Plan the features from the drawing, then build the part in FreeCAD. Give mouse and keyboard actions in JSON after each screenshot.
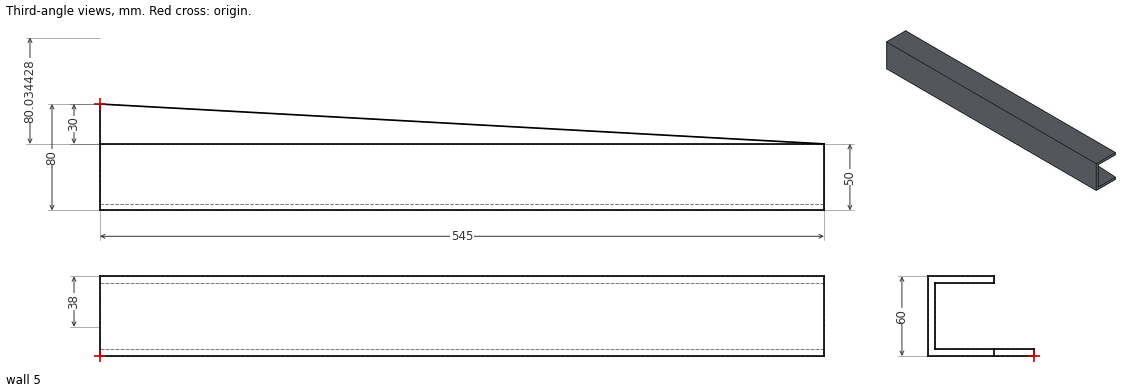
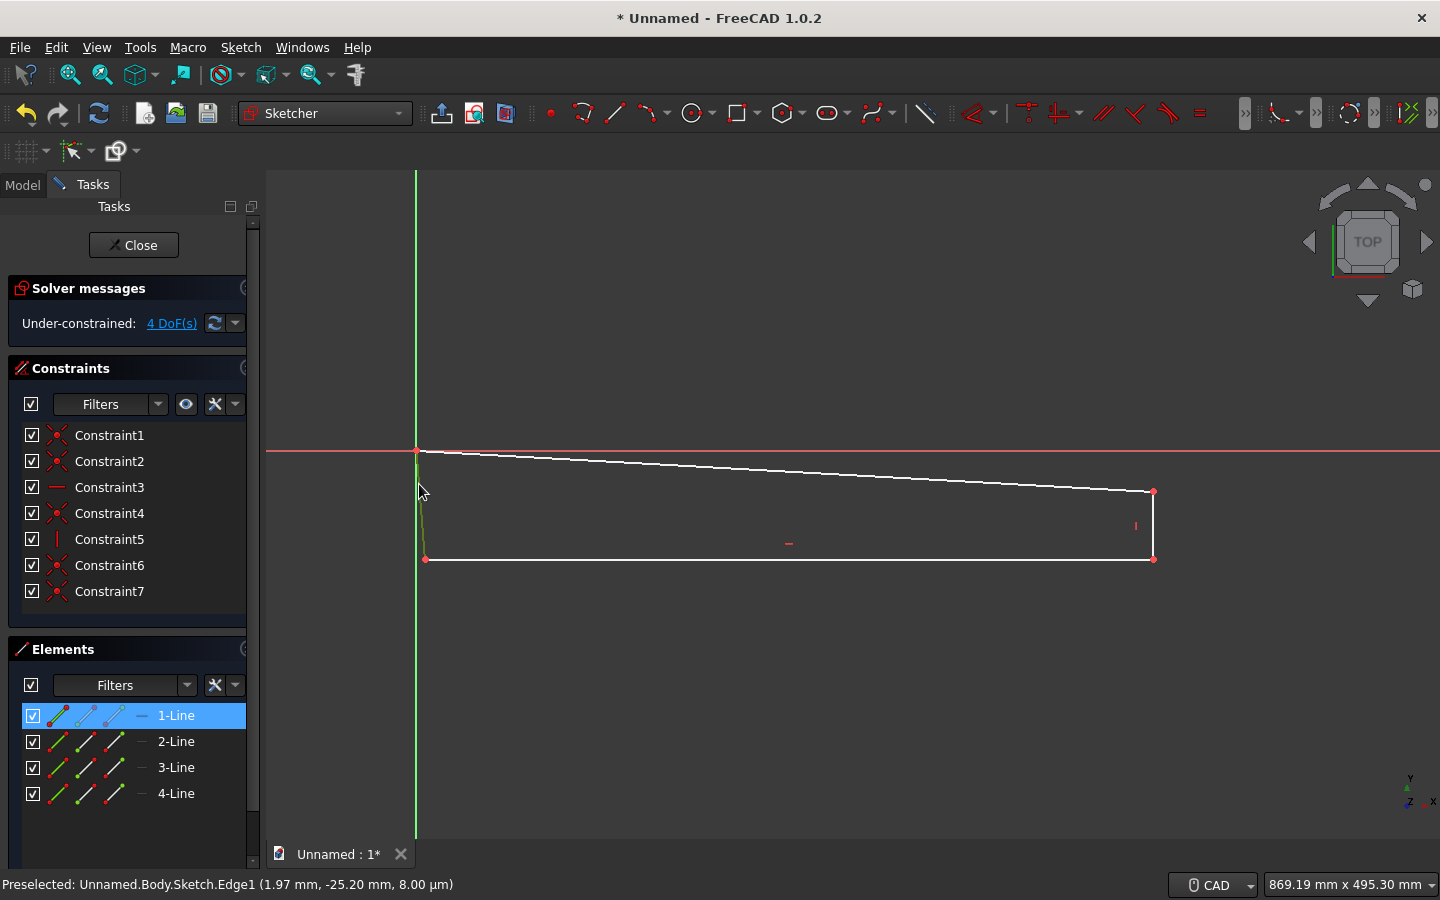
{"action": "key", "text": "v"}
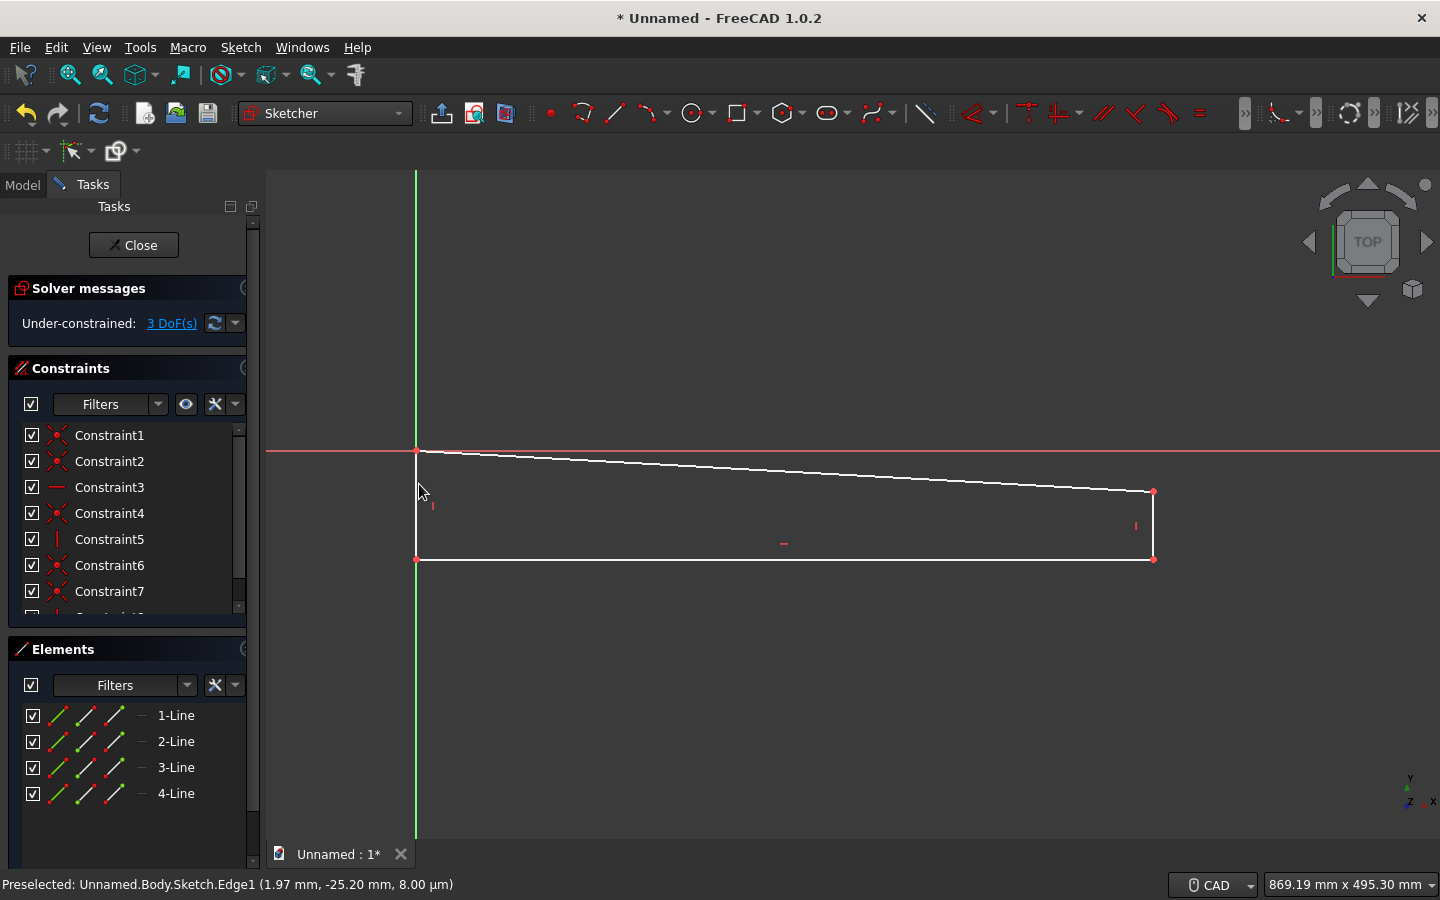
{"action": "left_click", "coordinate": [972, 114]}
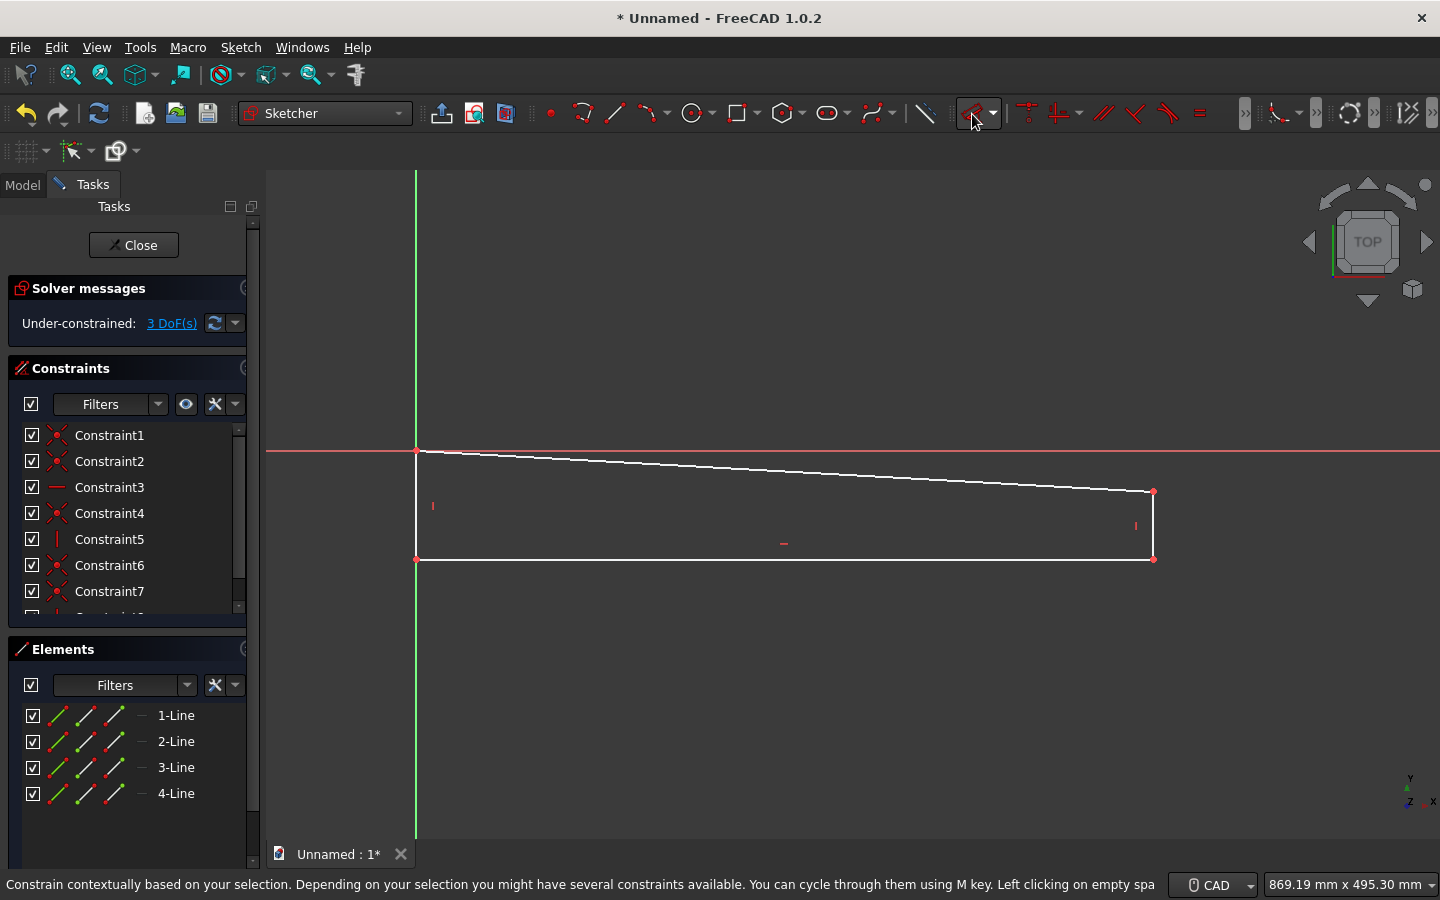
{"action": "left_click", "coordinate": [416, 484]}
{"action": "left_click", "coordinate": [382, 505]}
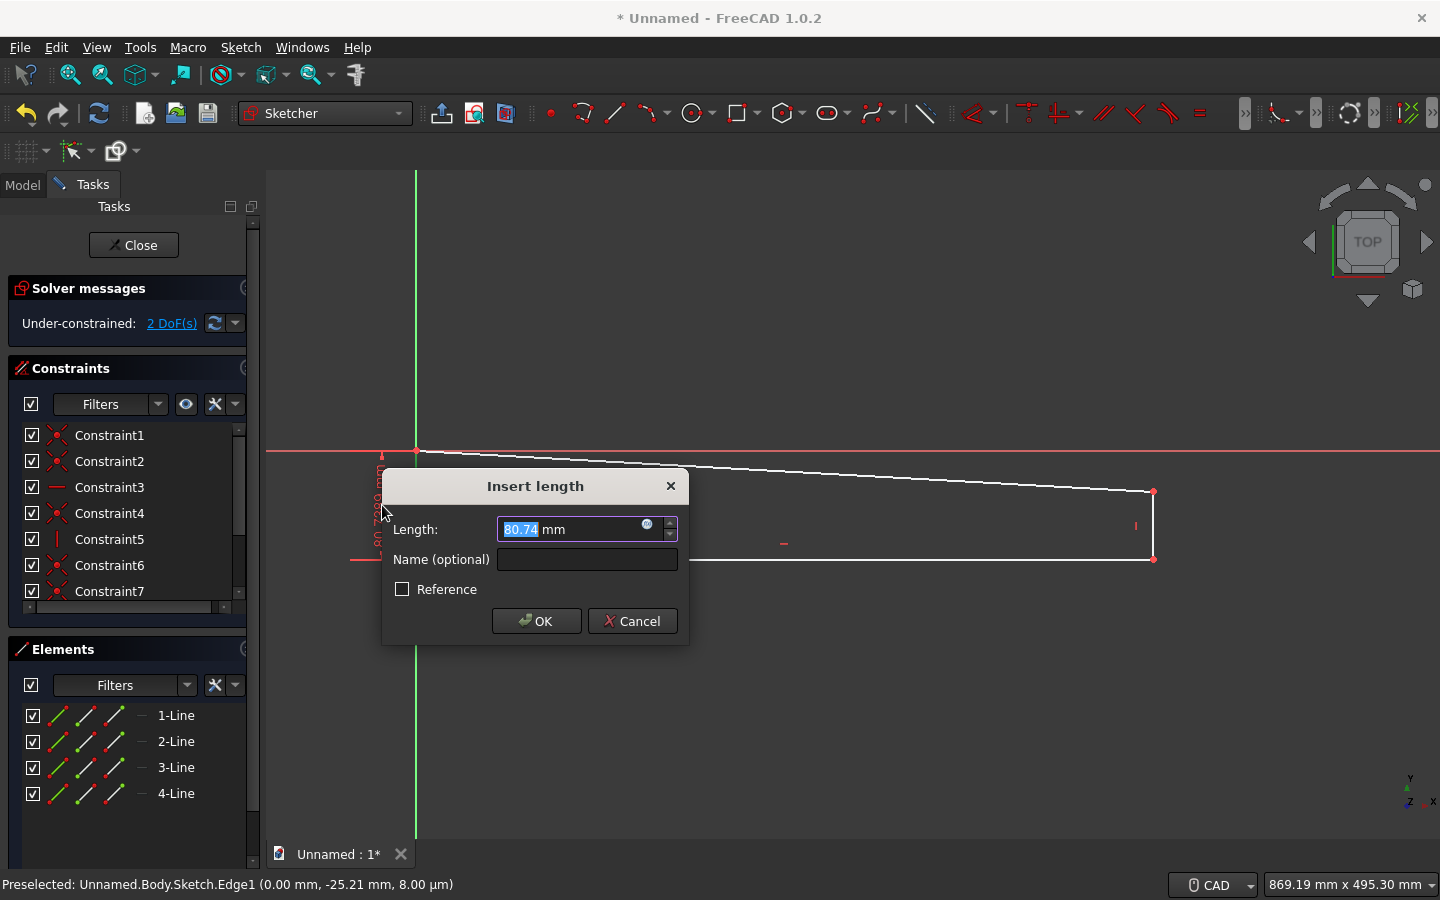
{"action": "type", "text": "80"}
{"action": "key", "text": "Return"}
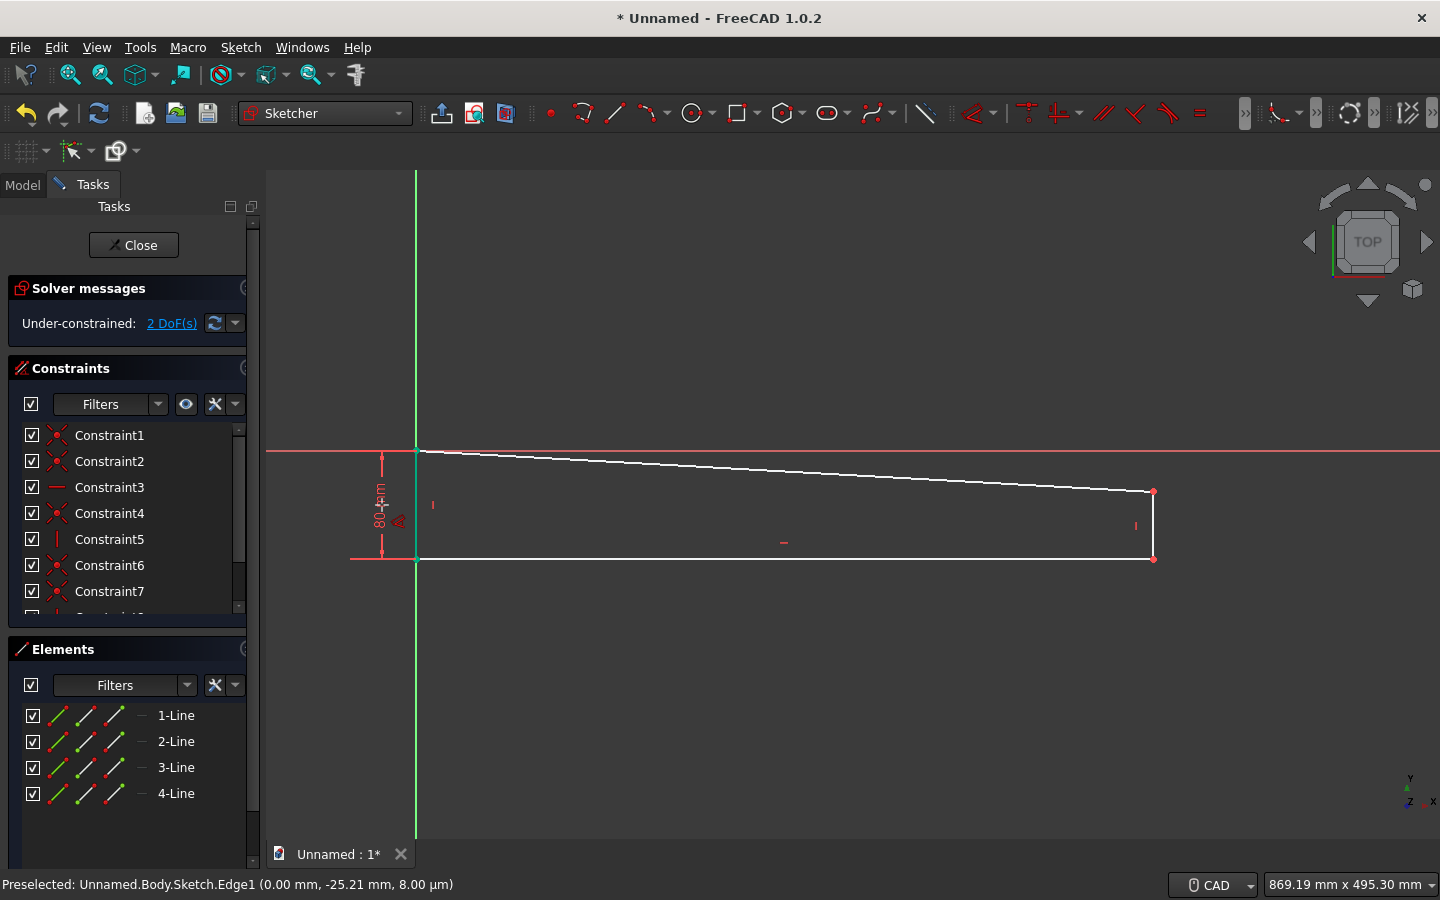
{"action": "left_click", "coordinate": [1153, 539]}
{"action": "left_click", "coordinate": [1187, 526]}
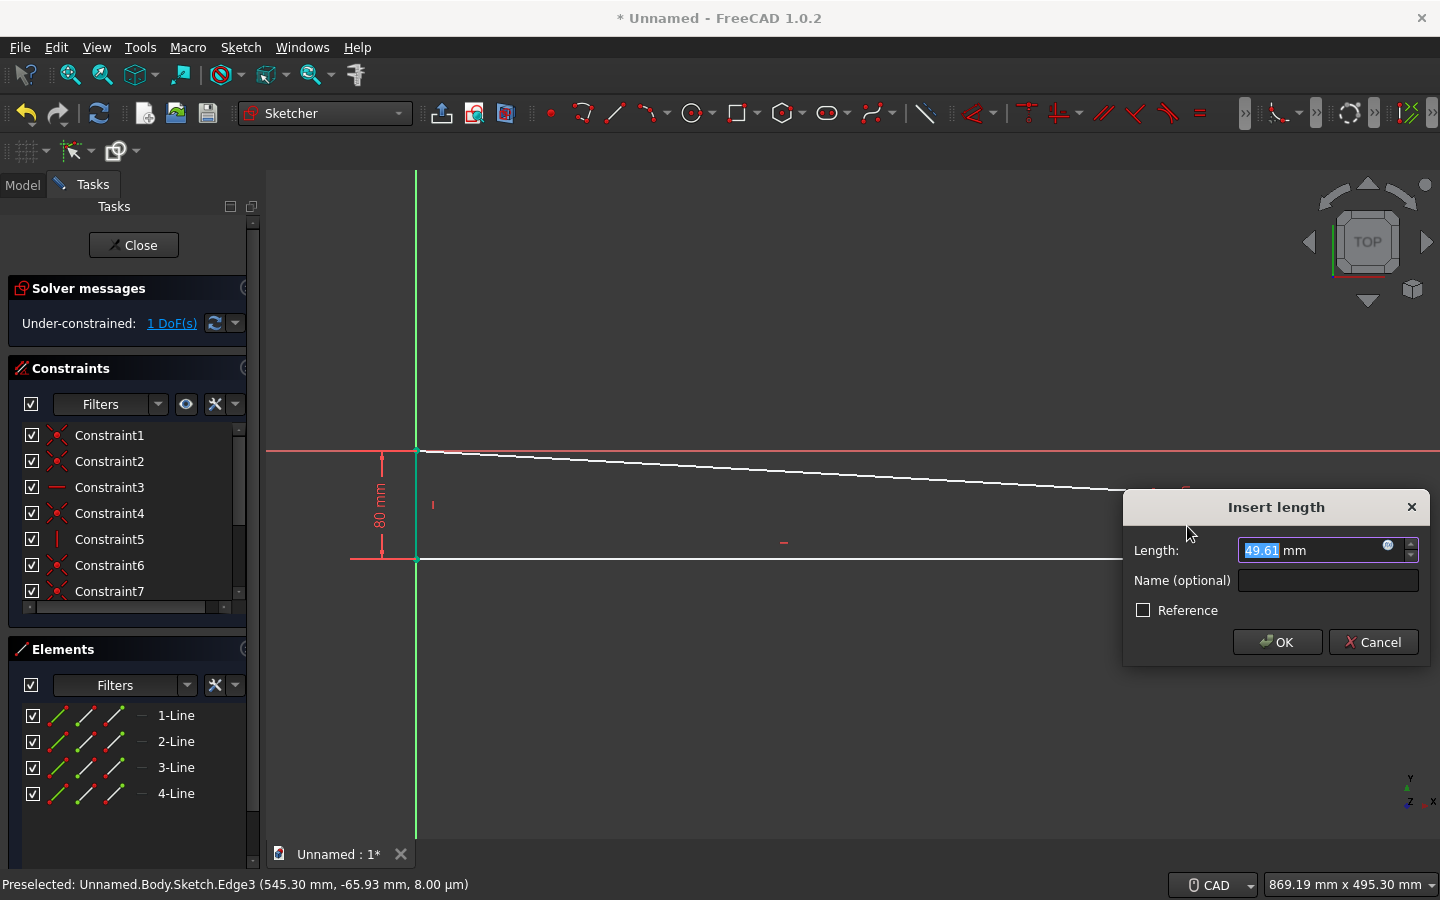
{"action": "type", "text": "50"}
{"action": "key", "text": "Return"}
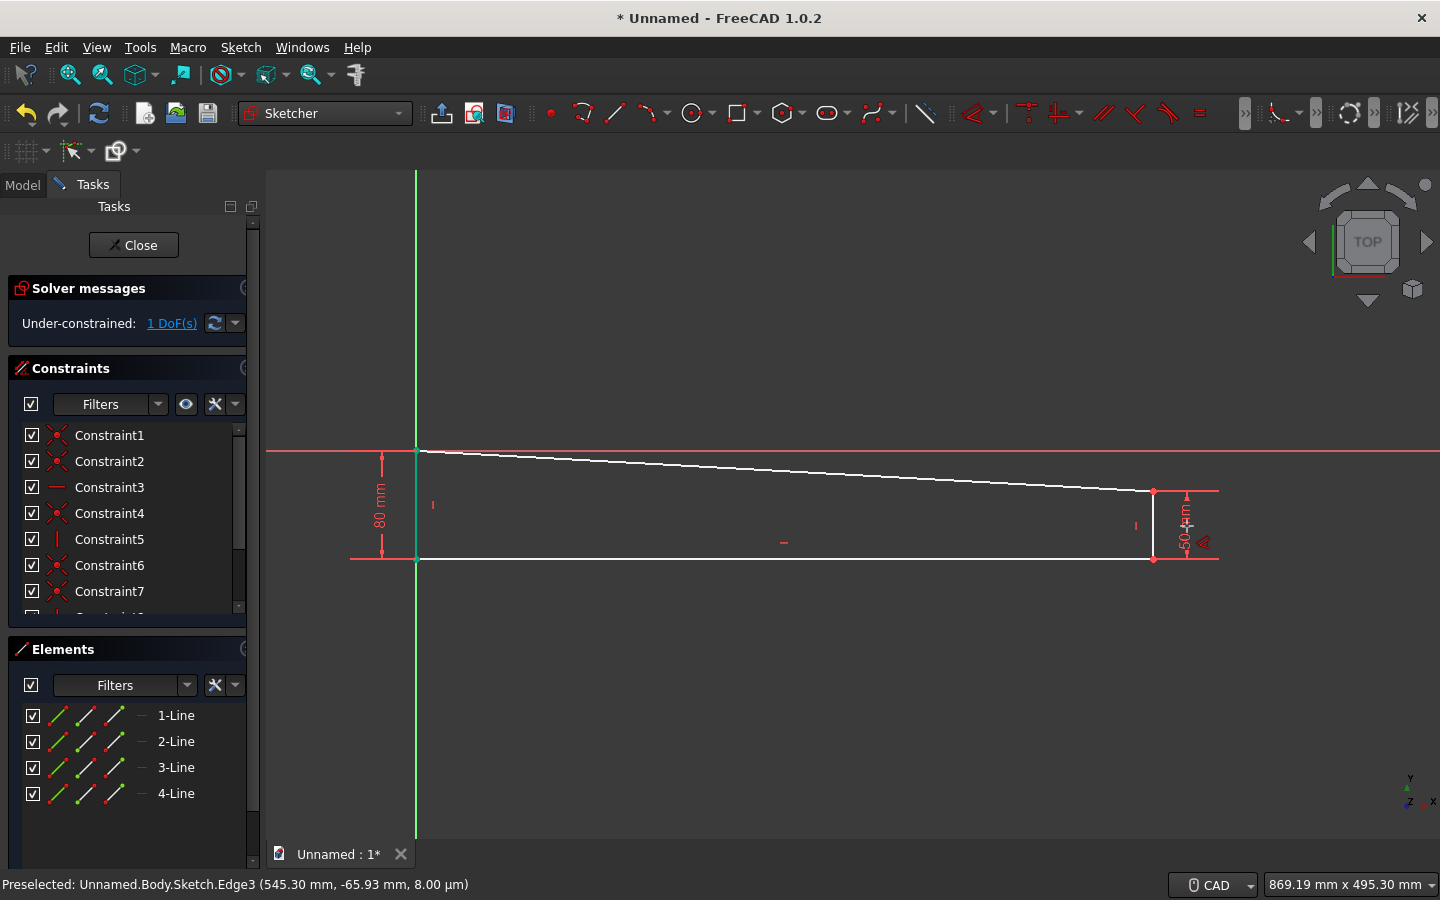
{"action": "left_click", "coordinate": [637, 559]}
{"action": "left_click", "coordinate": [785, 593]}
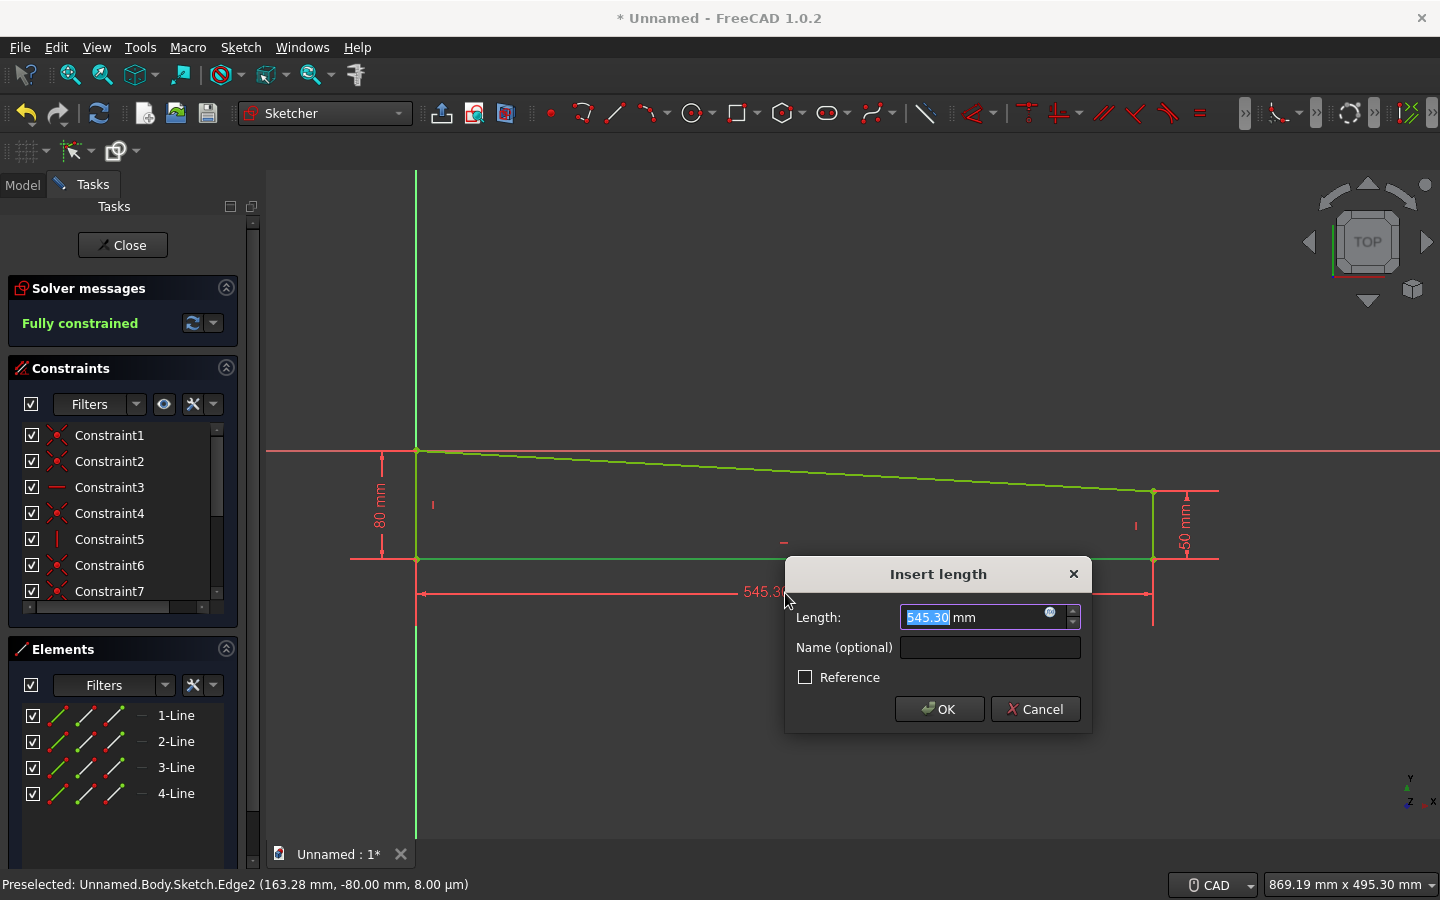
{"action": "type", "text": "545"}
{"action": "key", "text": "Return"}
{"action": "key", "text": "Escape"}